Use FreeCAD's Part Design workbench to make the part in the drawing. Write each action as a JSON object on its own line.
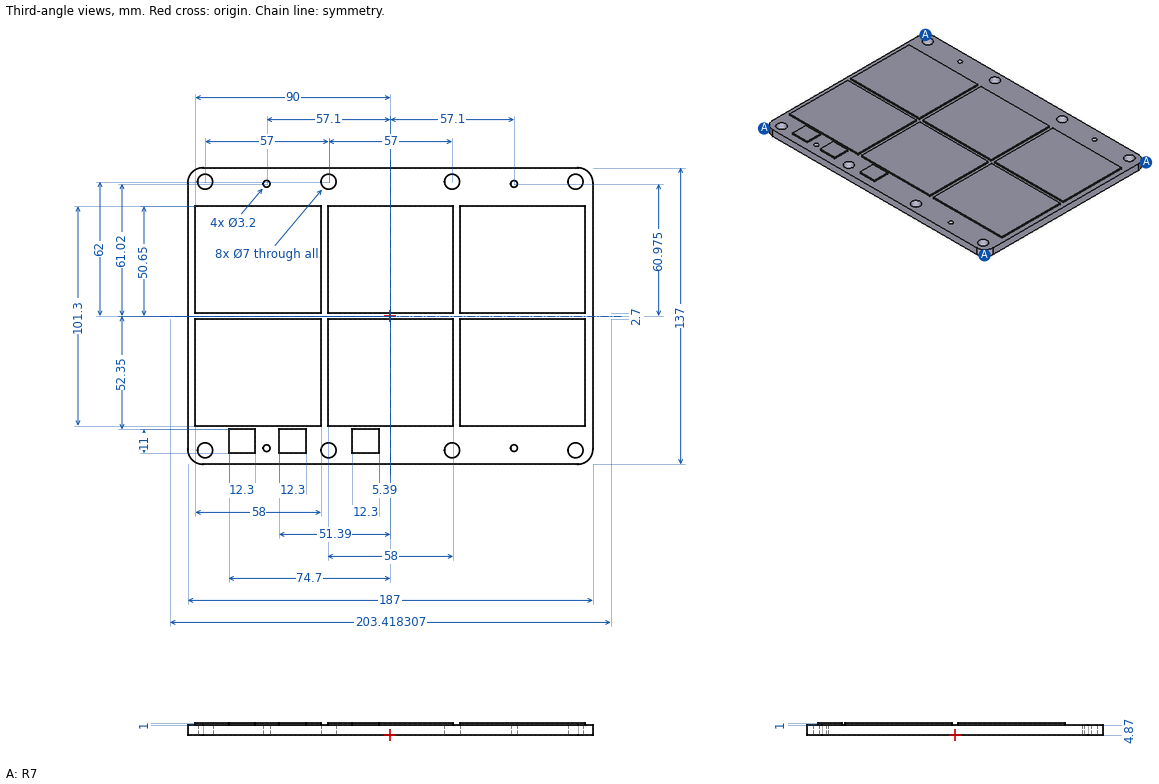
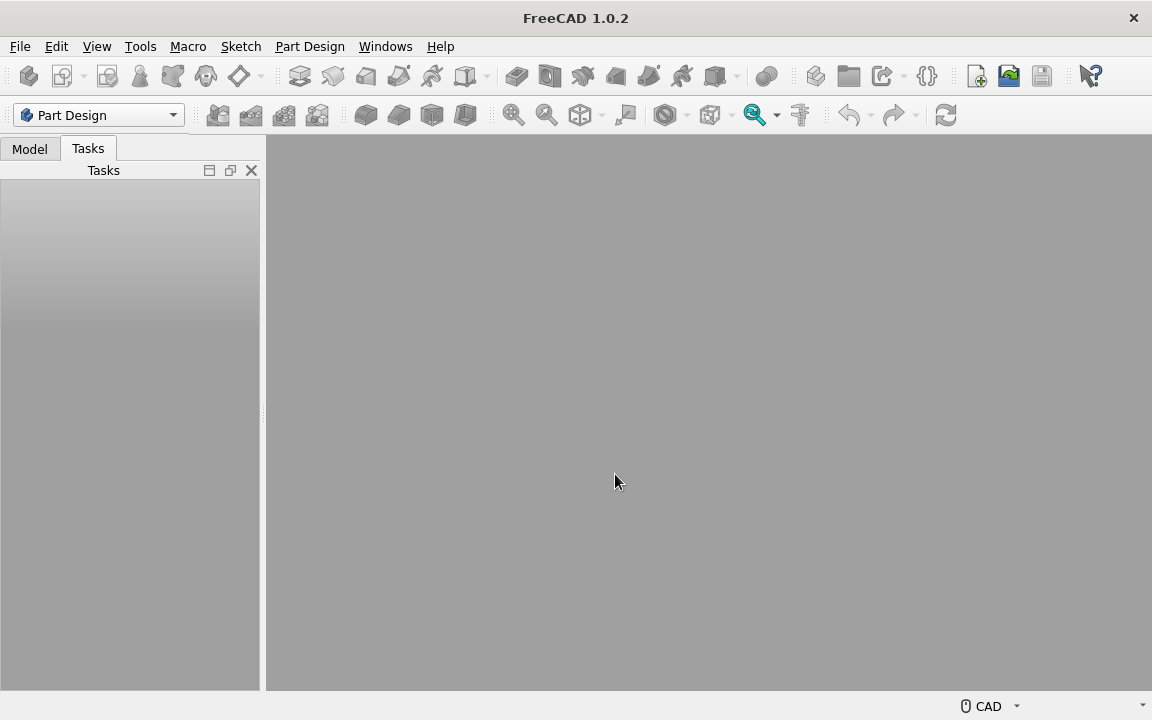
{"action": "key", "text": "ctrl+n"}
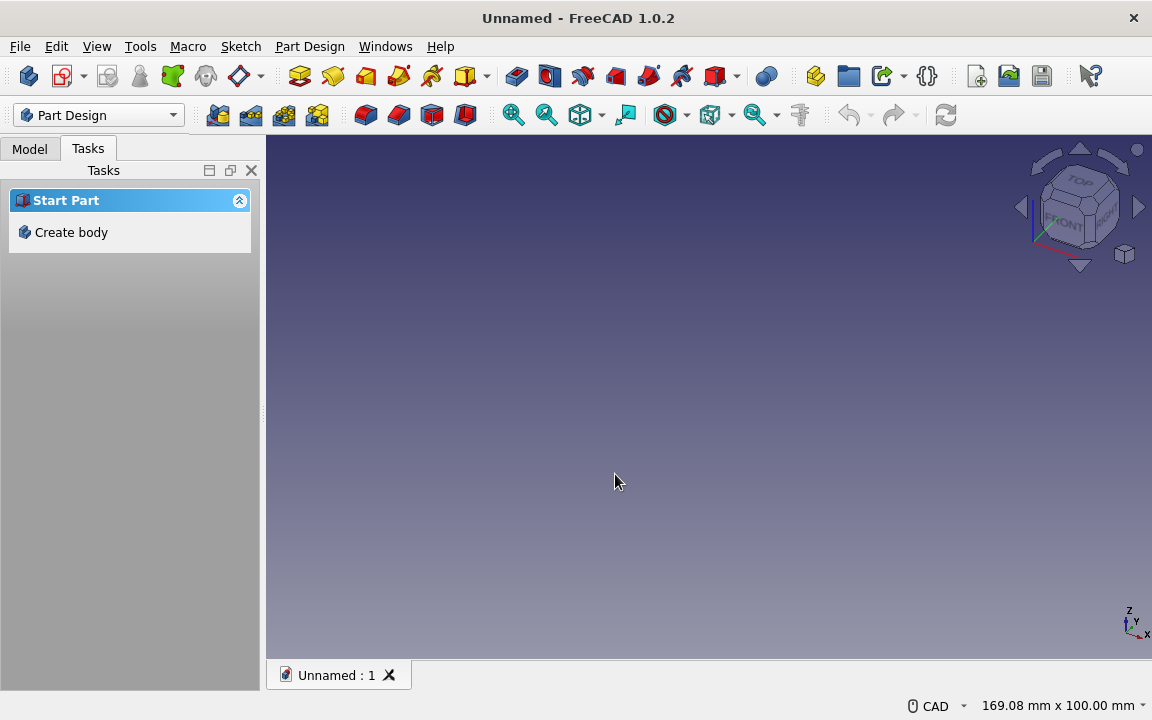
{"action": "left_click", "coordinate": [62, 76]}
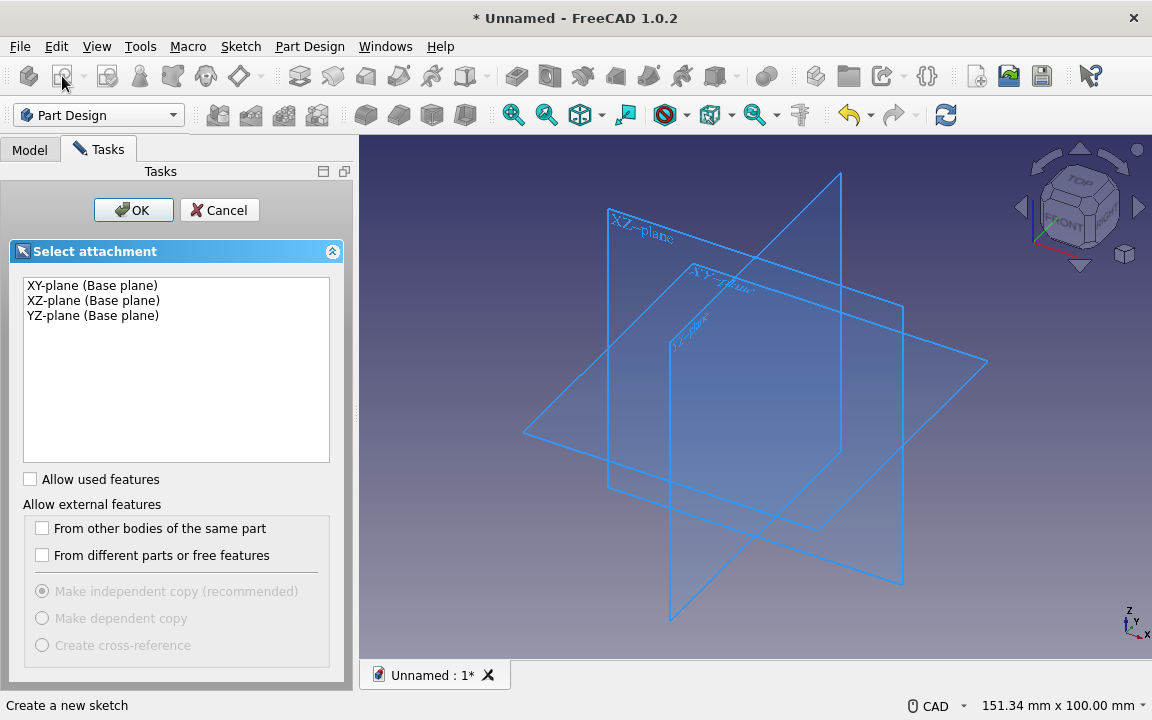
{"action": "left_click", "coordinate": [84, 286]}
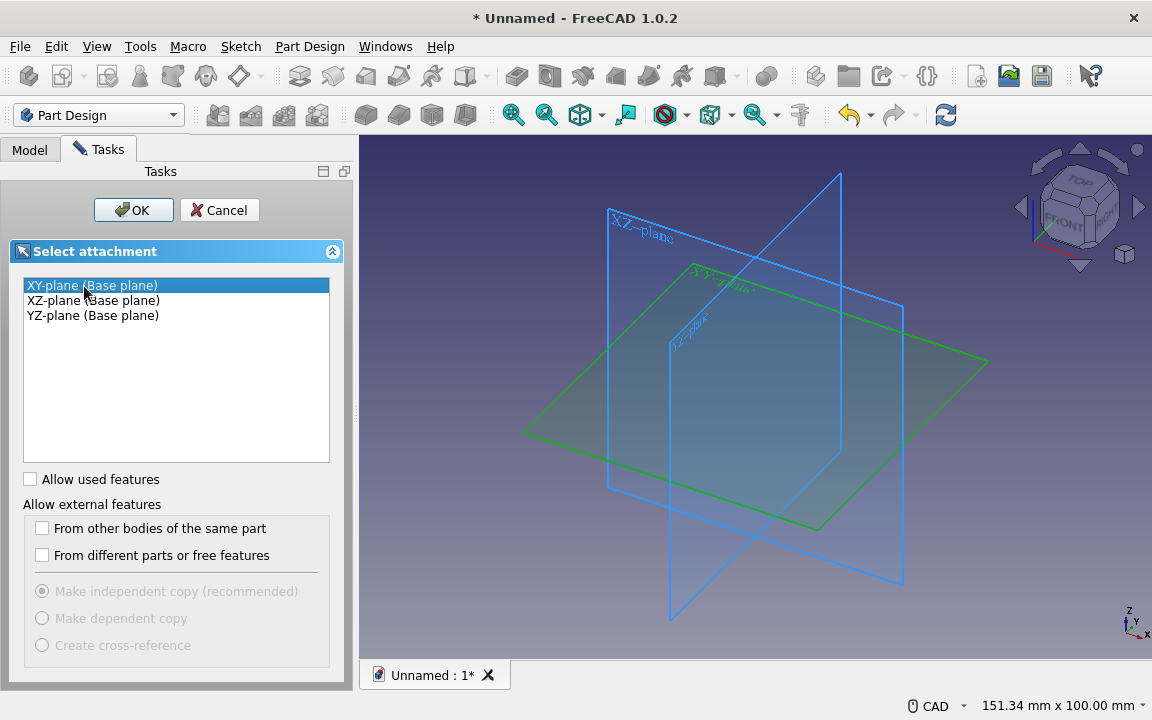
{"action": "left_click", "coordinate": [134, 210]}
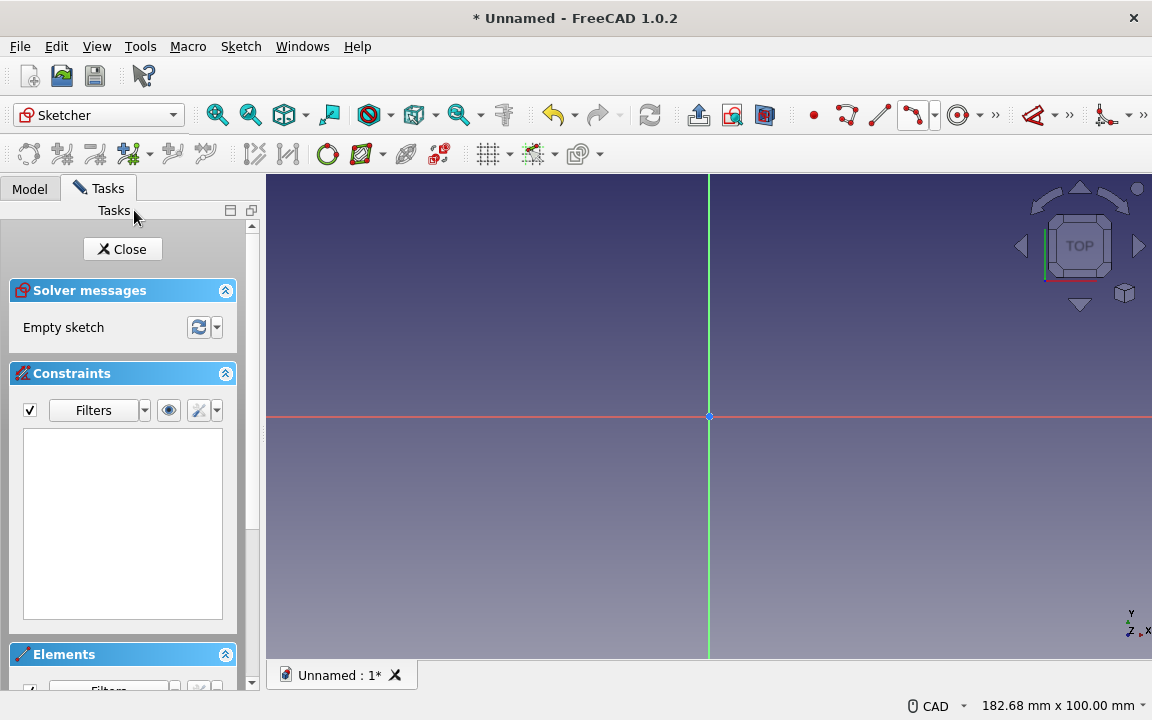
{"action": "scroll", "coordinate": [585, 416], "scroll_direction": "down", "scroll_amount": 4}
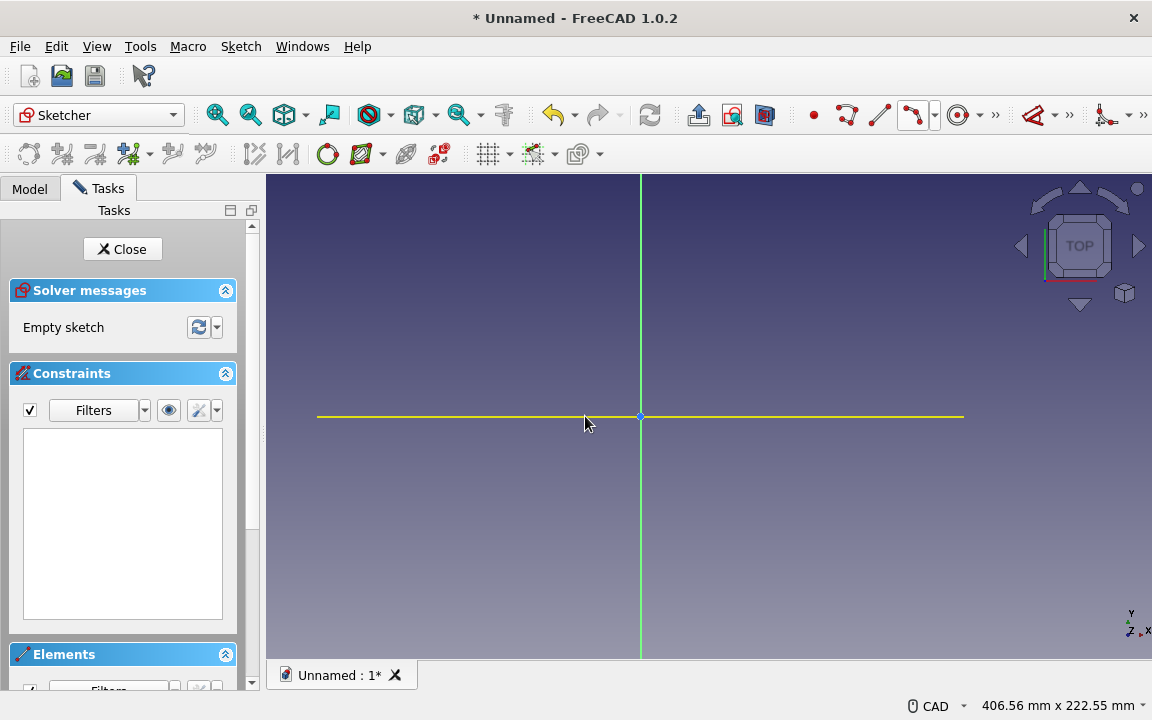
{"action": "key", "text": "g v"}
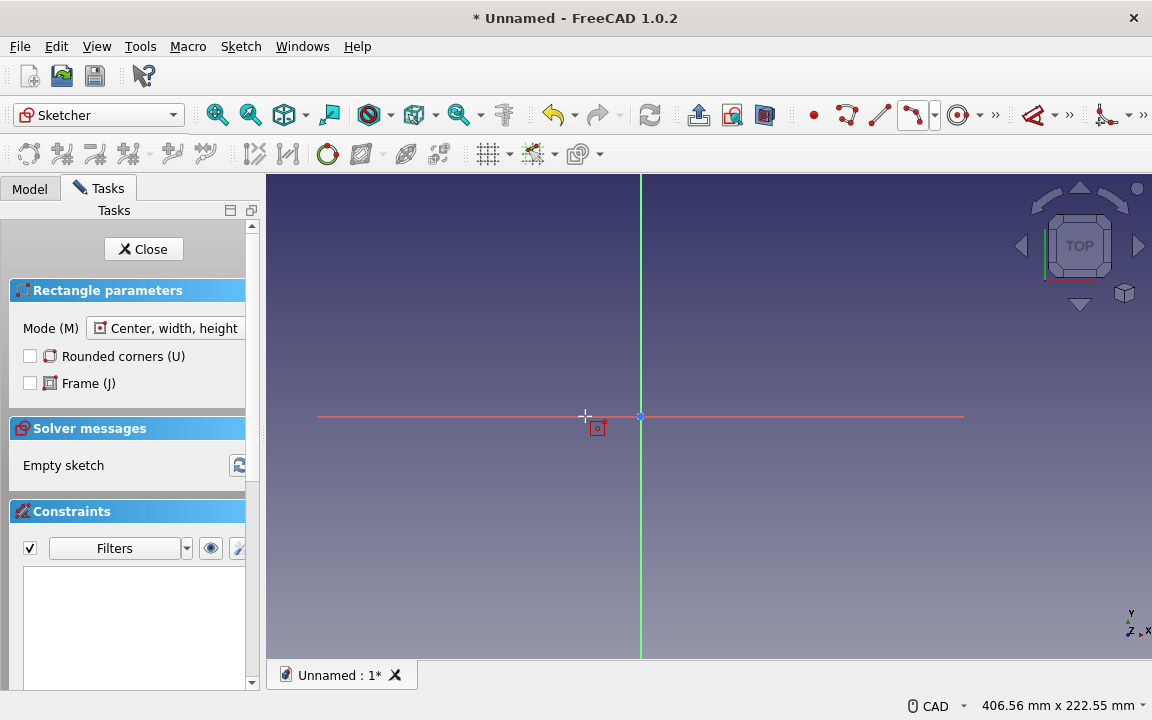
{"action": "left_click", "coordinate": [641, 416]}
{"action": "left_click", "coordinate": [845, 267]}
{"action": "key", "text": "Escape"}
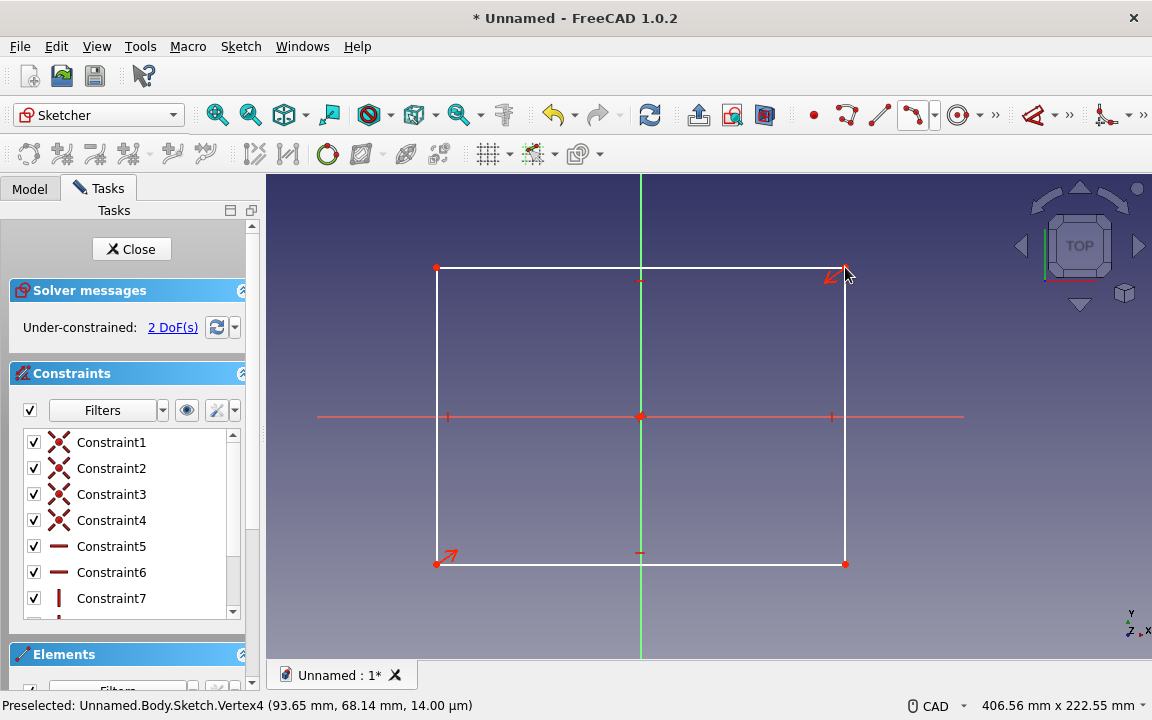
{"action": "left_click", "coordinate": [1032, 116]}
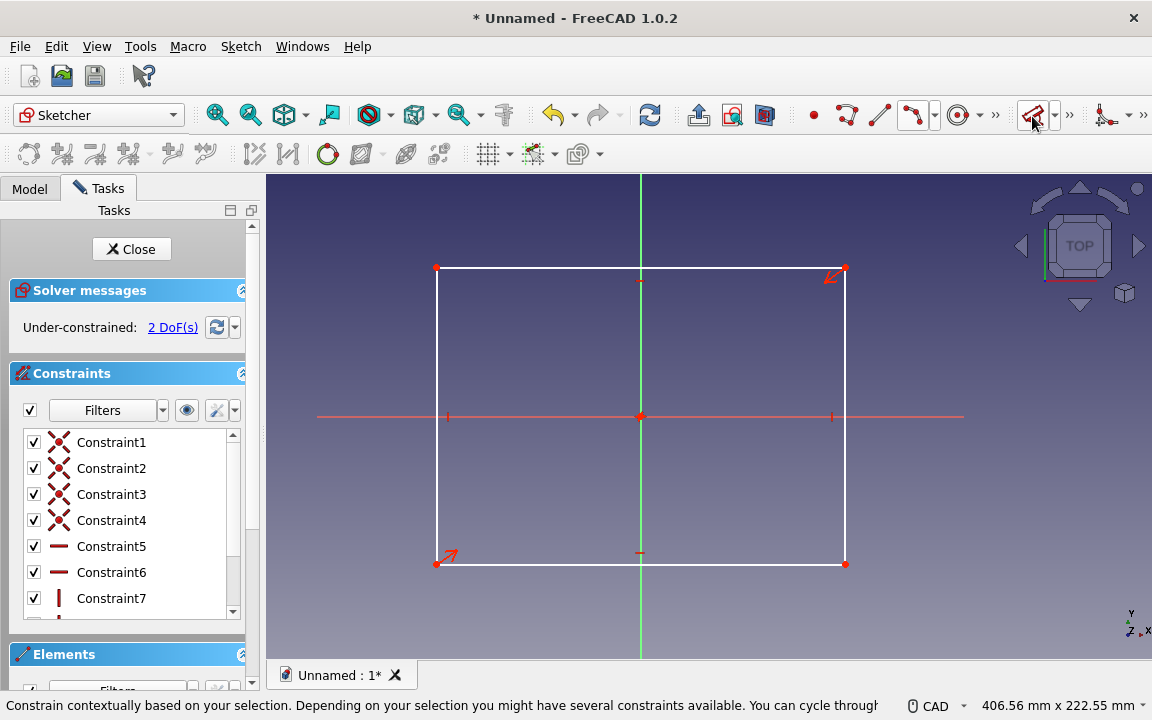
{"action": "left_click", "coordinate": [559, 565]}
{"action": "left_click", "coordinate": [547, 599]}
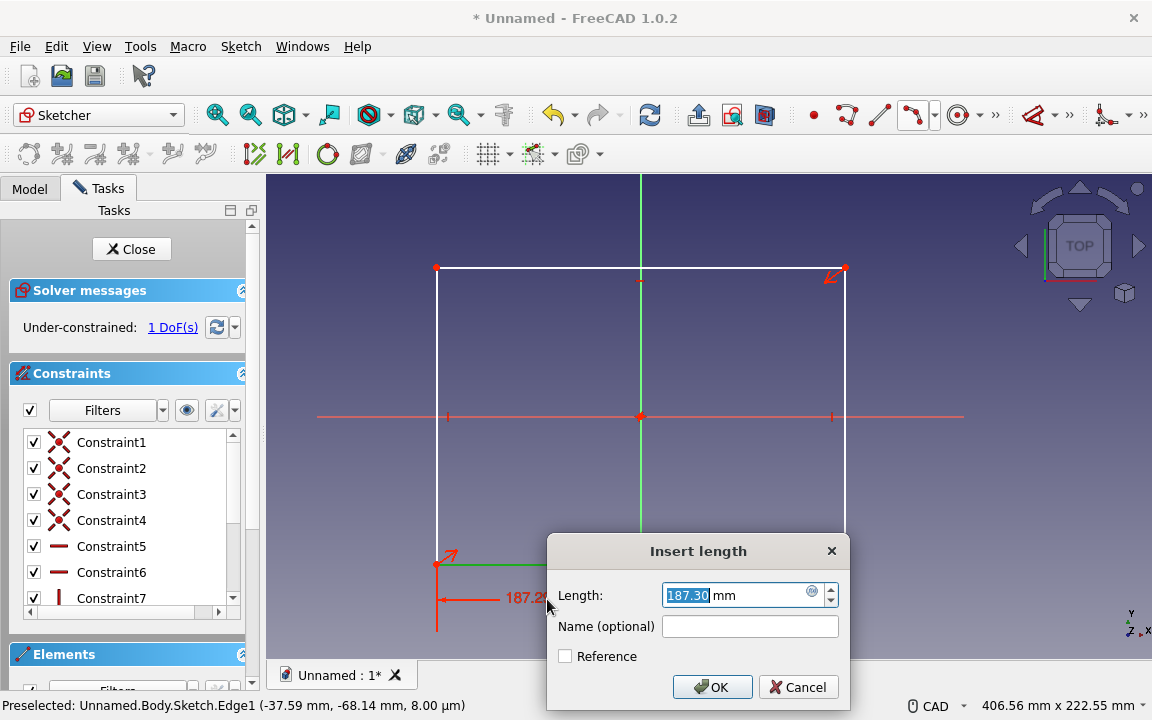
{"action": "type", "text": "187"}
{"action": "key", "text": "Return"}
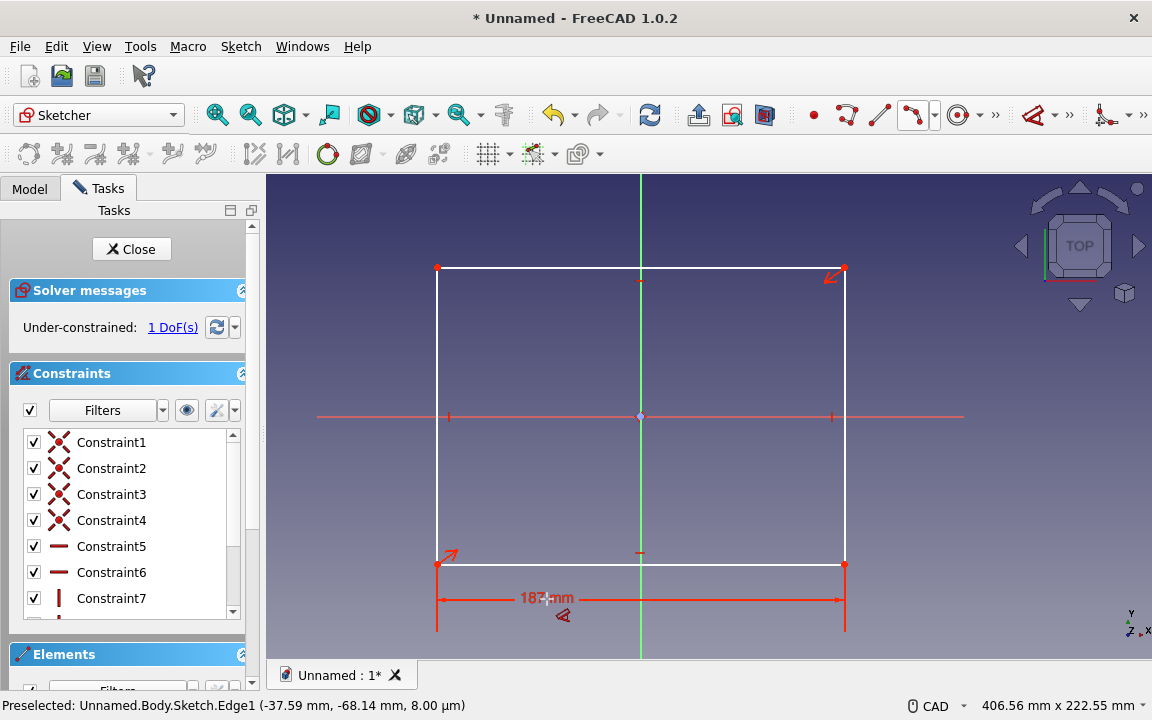
{"action": "left_click", "coordinate": [845, 476]}
{"action": "left_click", "coordinate": [879, 348]}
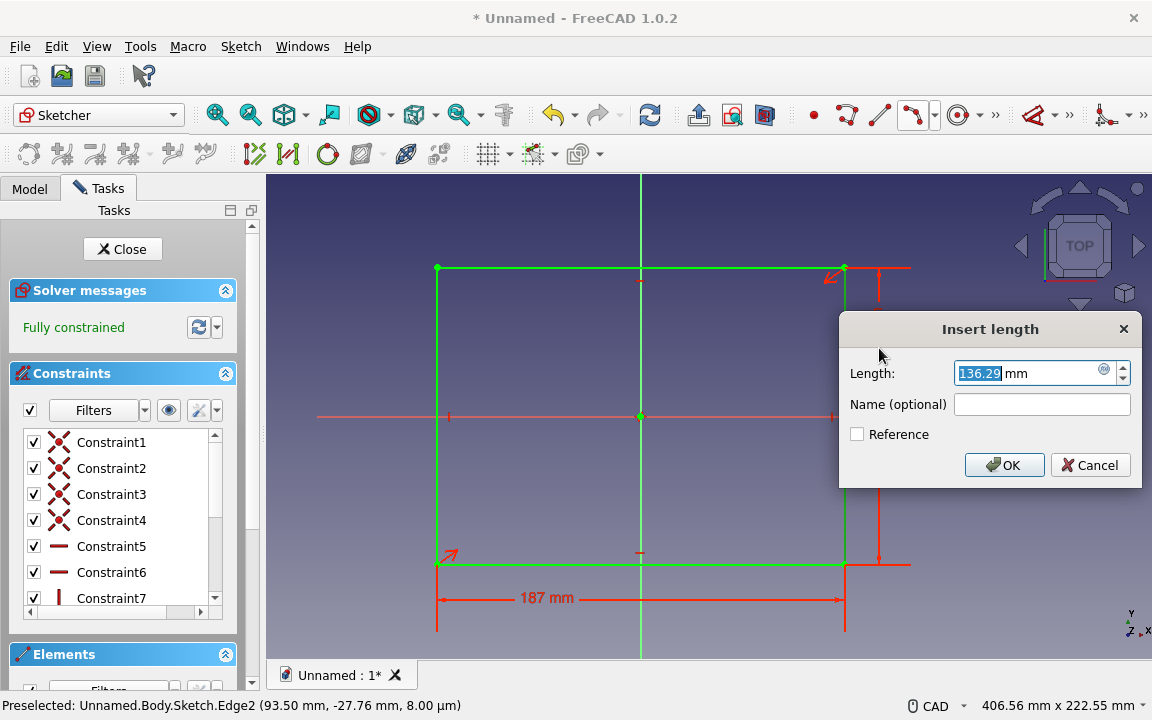
{"action": "type", "text": "137"}
{"action": "key", "text": "Return"}
{"action": "key", "text": "Escape"}